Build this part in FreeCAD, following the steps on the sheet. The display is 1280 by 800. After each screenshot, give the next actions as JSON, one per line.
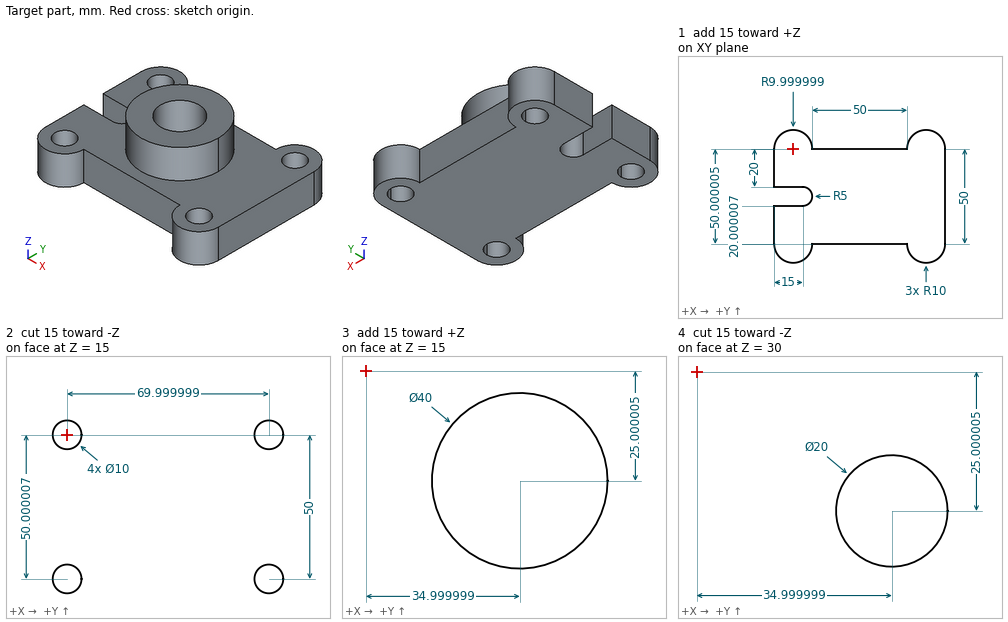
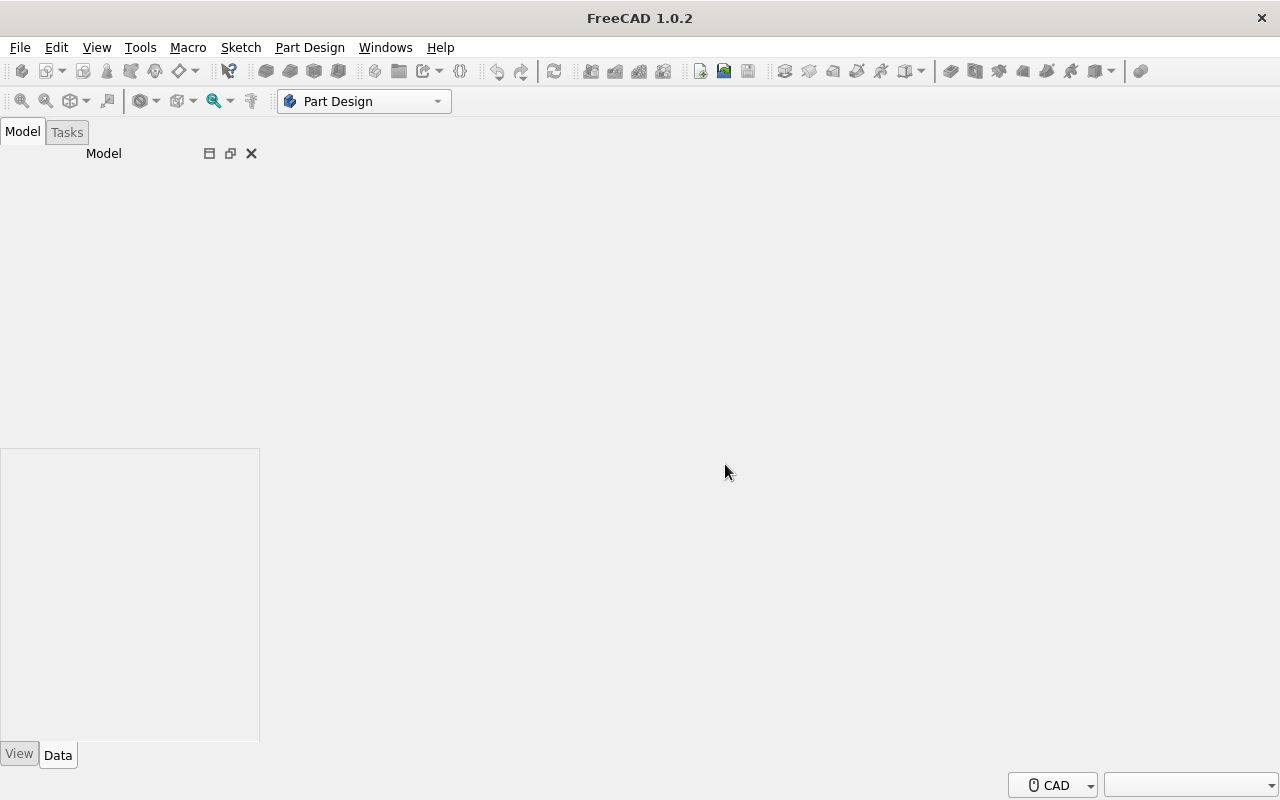
{"action": "left_click", "coordinate": [700, 72]}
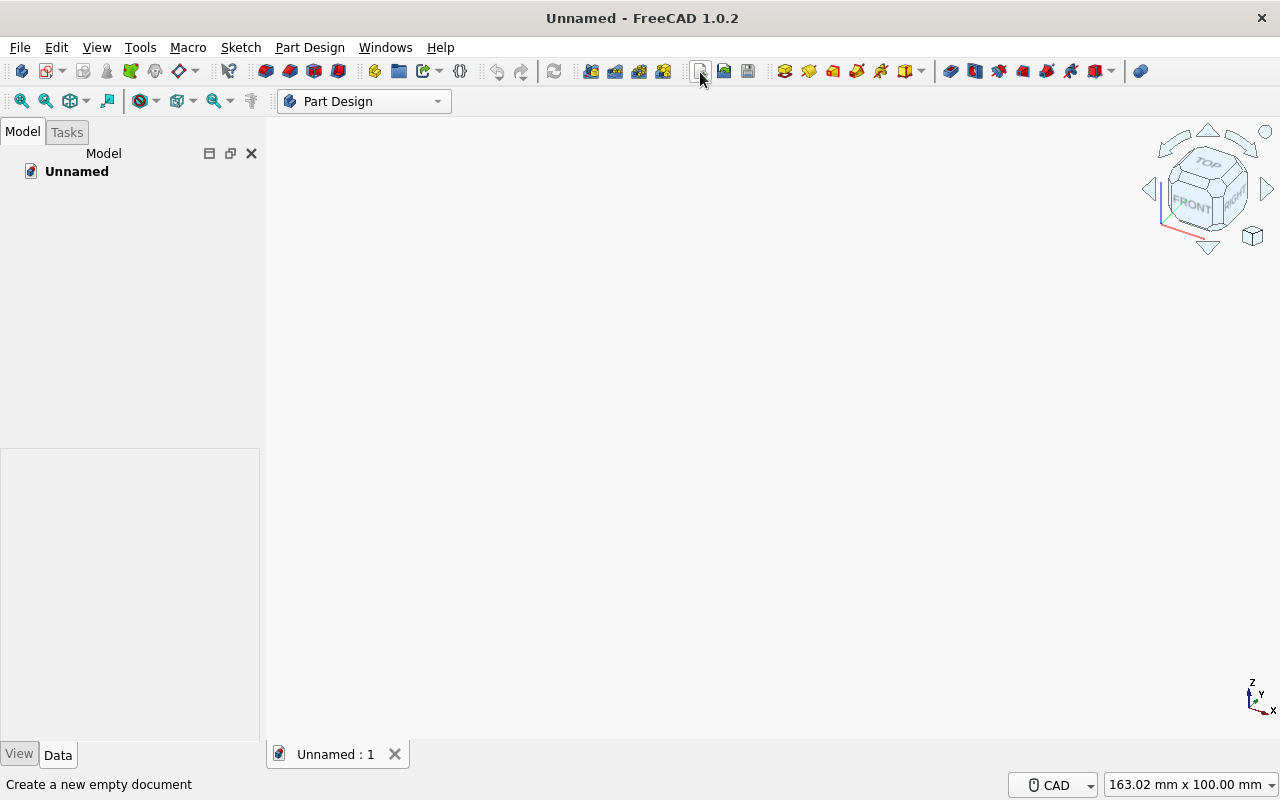
{"action": "left_click", "coordinate": [46, 72]}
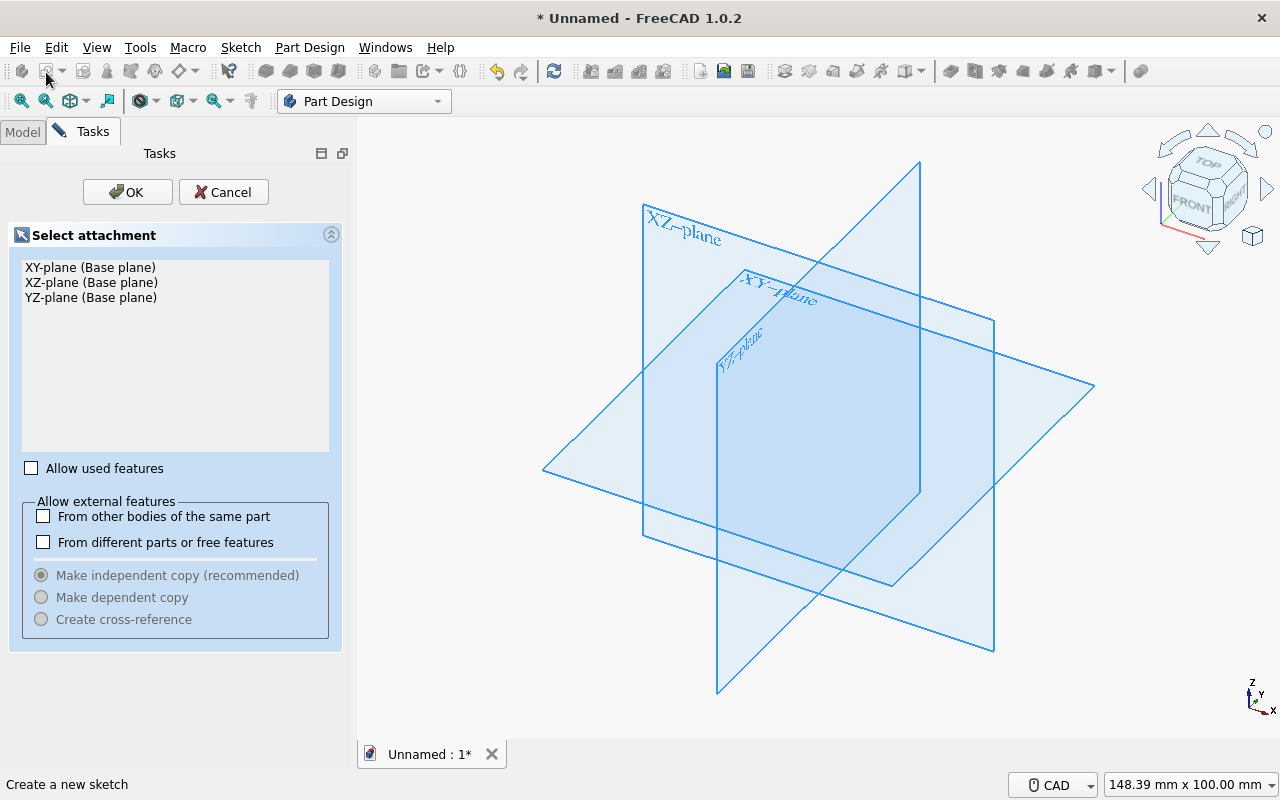
{"action": "left_click", "coordinate": [82, 268]}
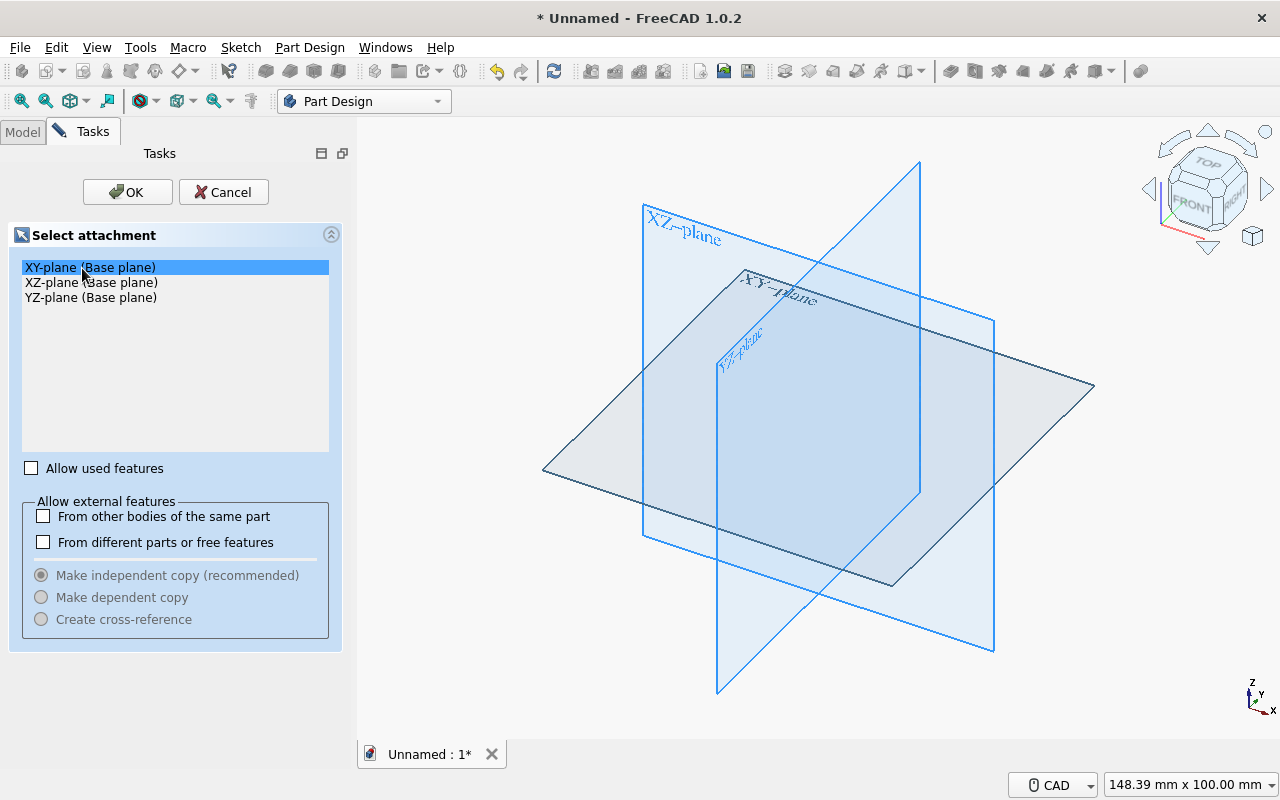
{"action": "left_click", "coordinate": [128, 192]}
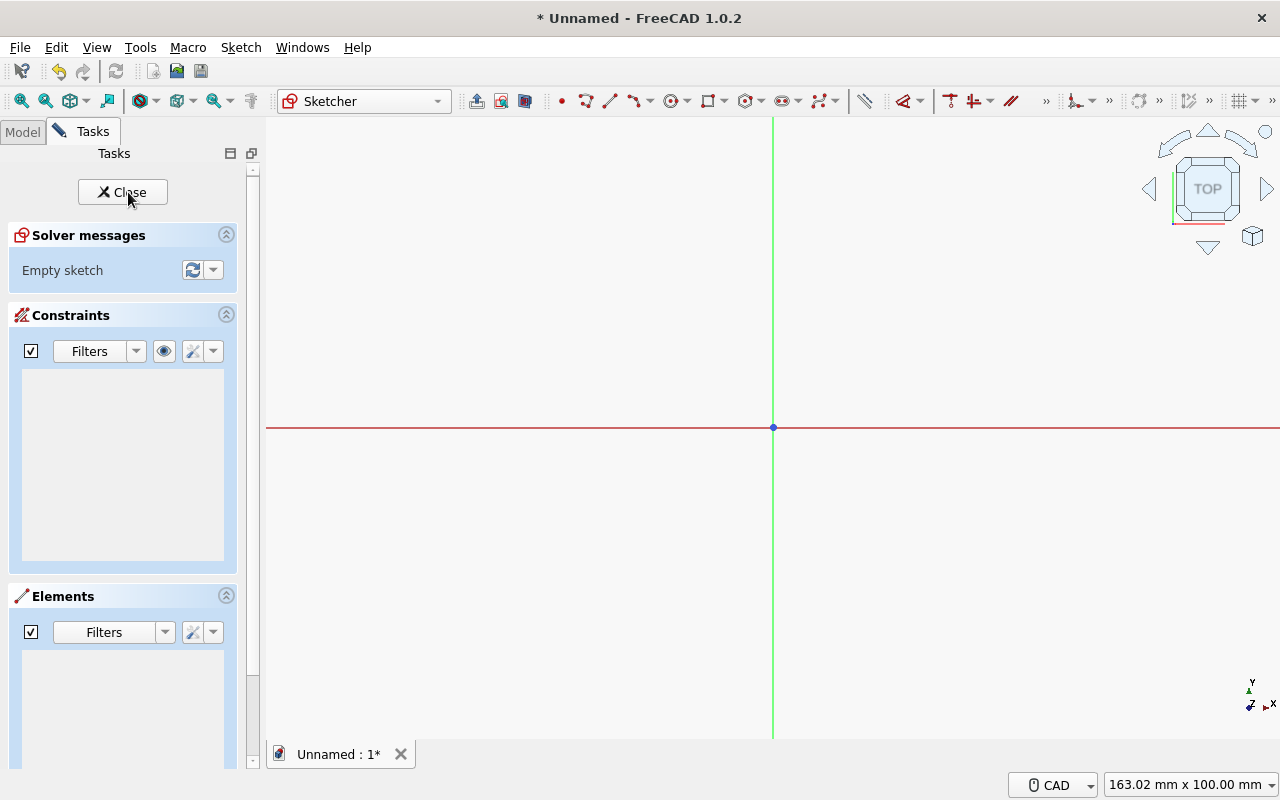
{"action": "scroll", "coordinate": [294, 145], "scroll_direction": "down", "scroll_amount": 2}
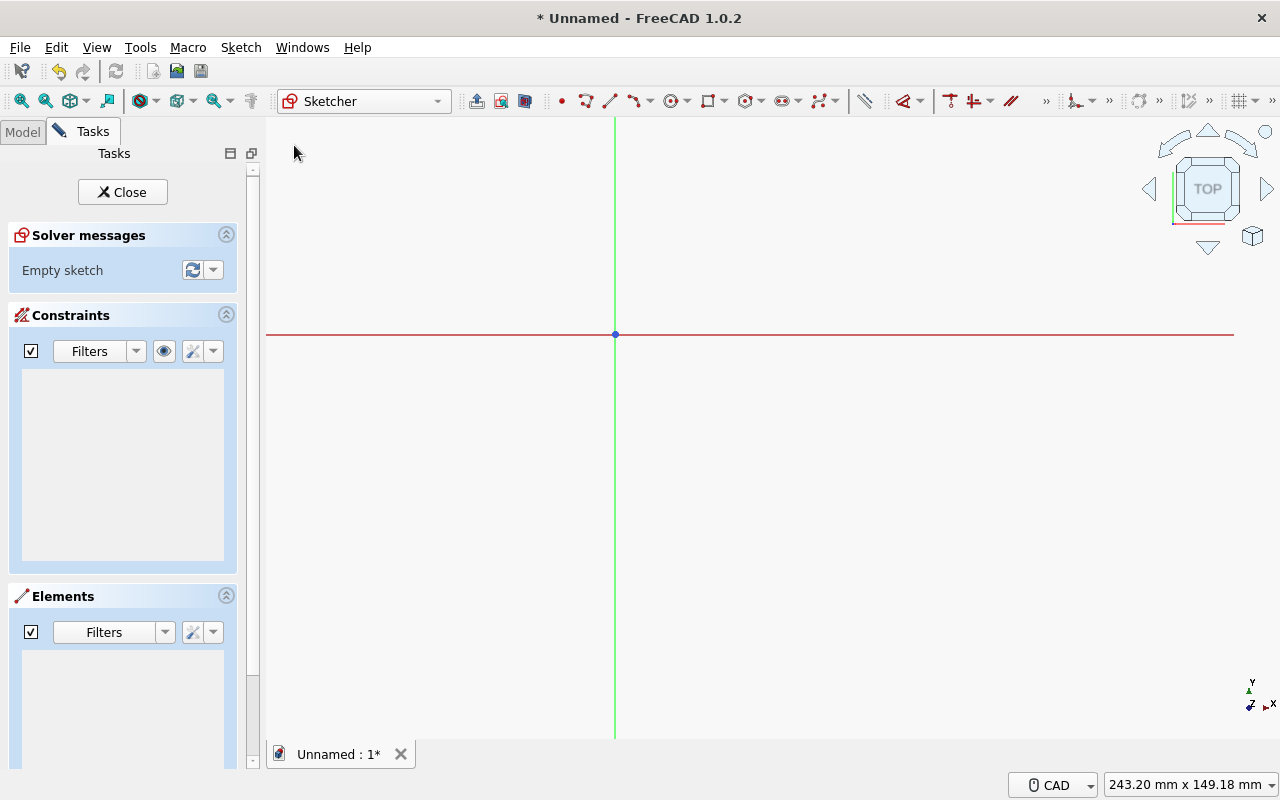
{"action": "scroll", "coordinate": [876, 461], "scroll_direction": "up", "scroll_amount": 2}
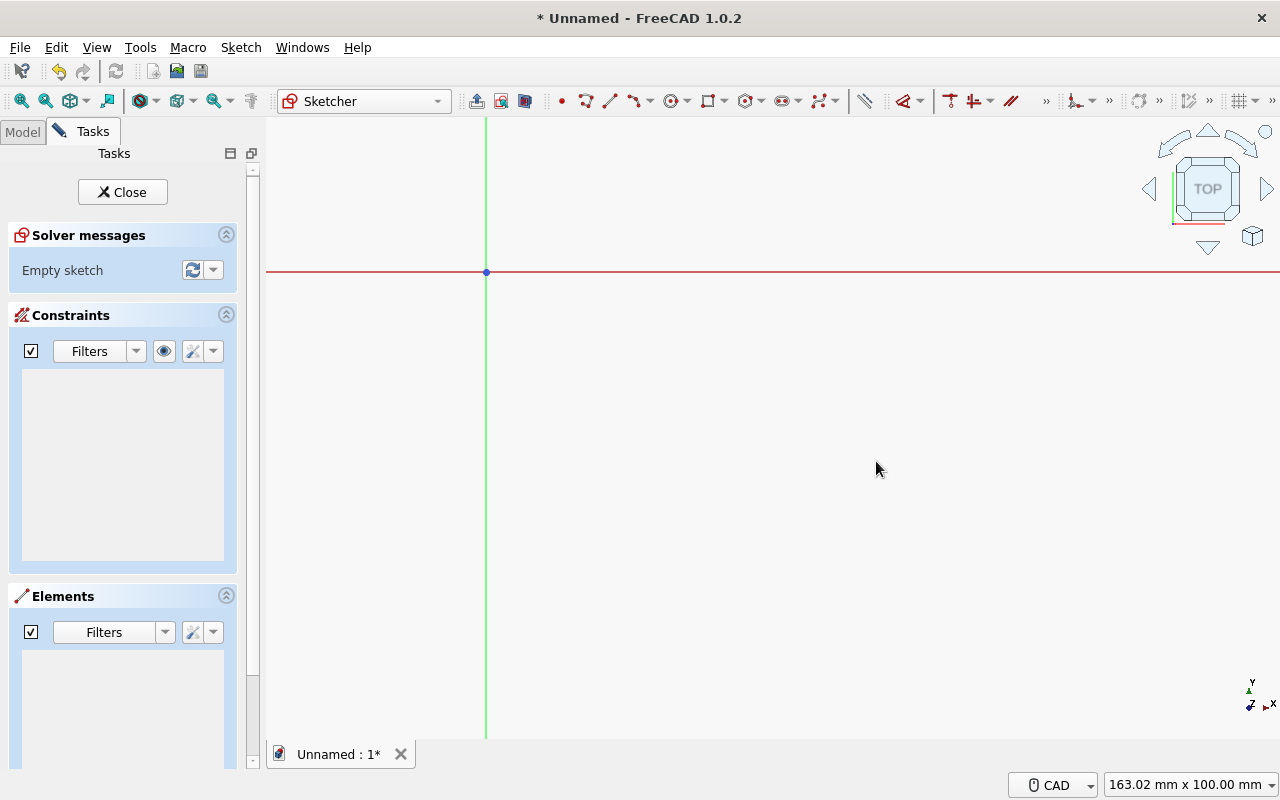
{"action": "left_click", "coordinate": [610, 102]}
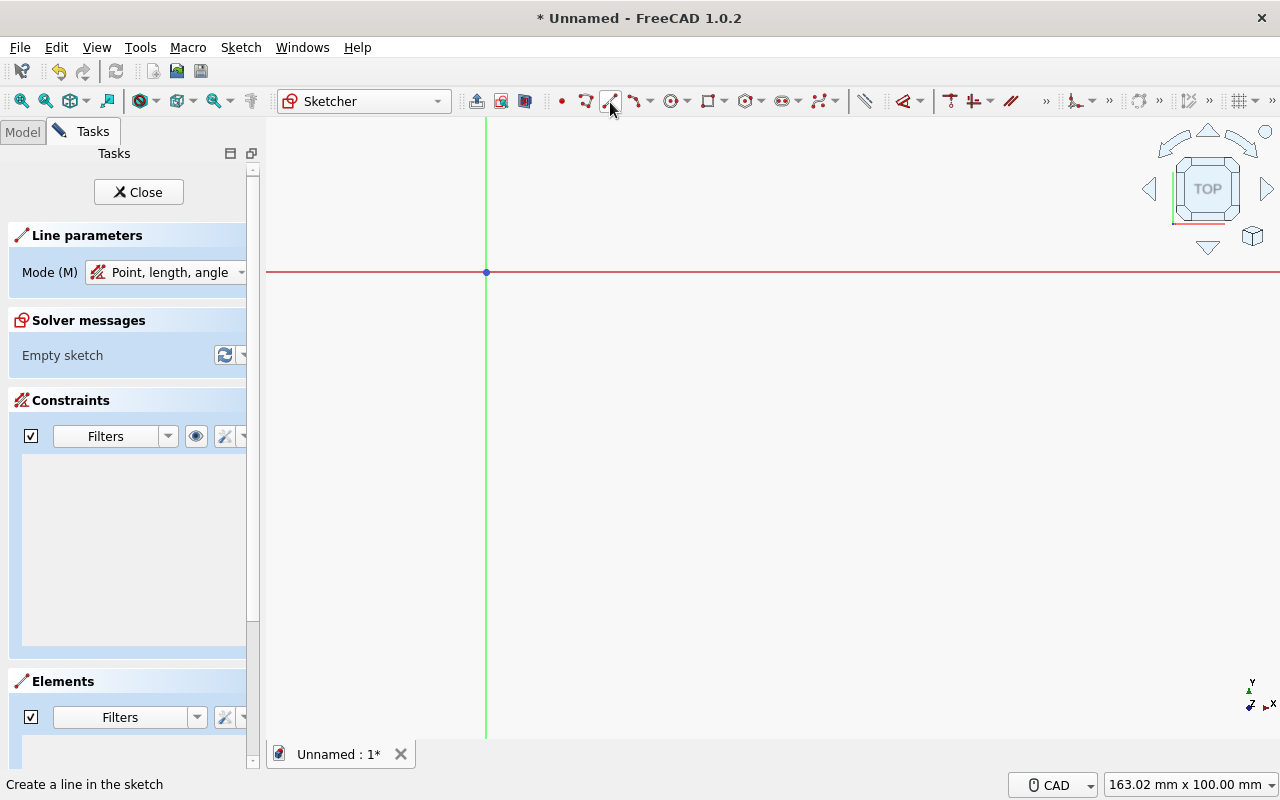
{"action": "left_click", "coordinate": [860, 272]}
{"action": "left_click", "coordinate": [549, 281]}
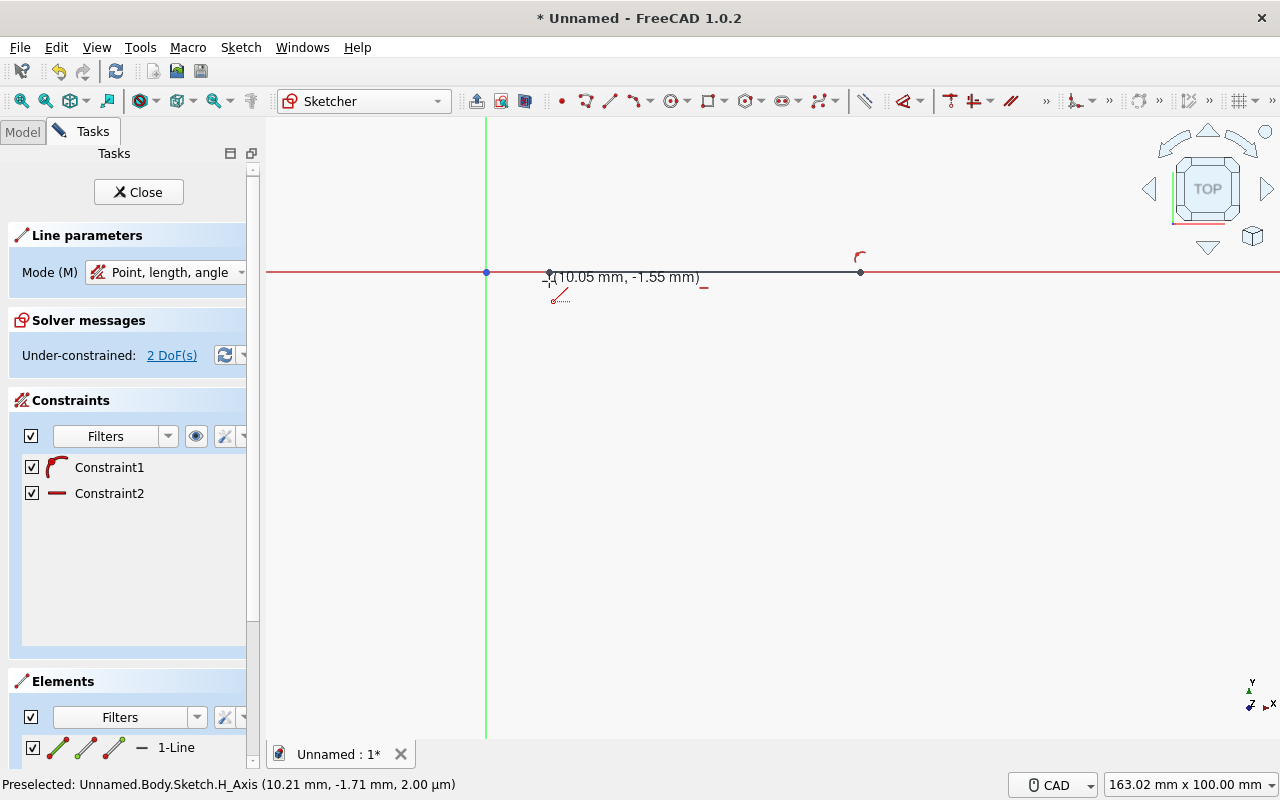
{"action": "left_click", "coordinate": [586, 102]}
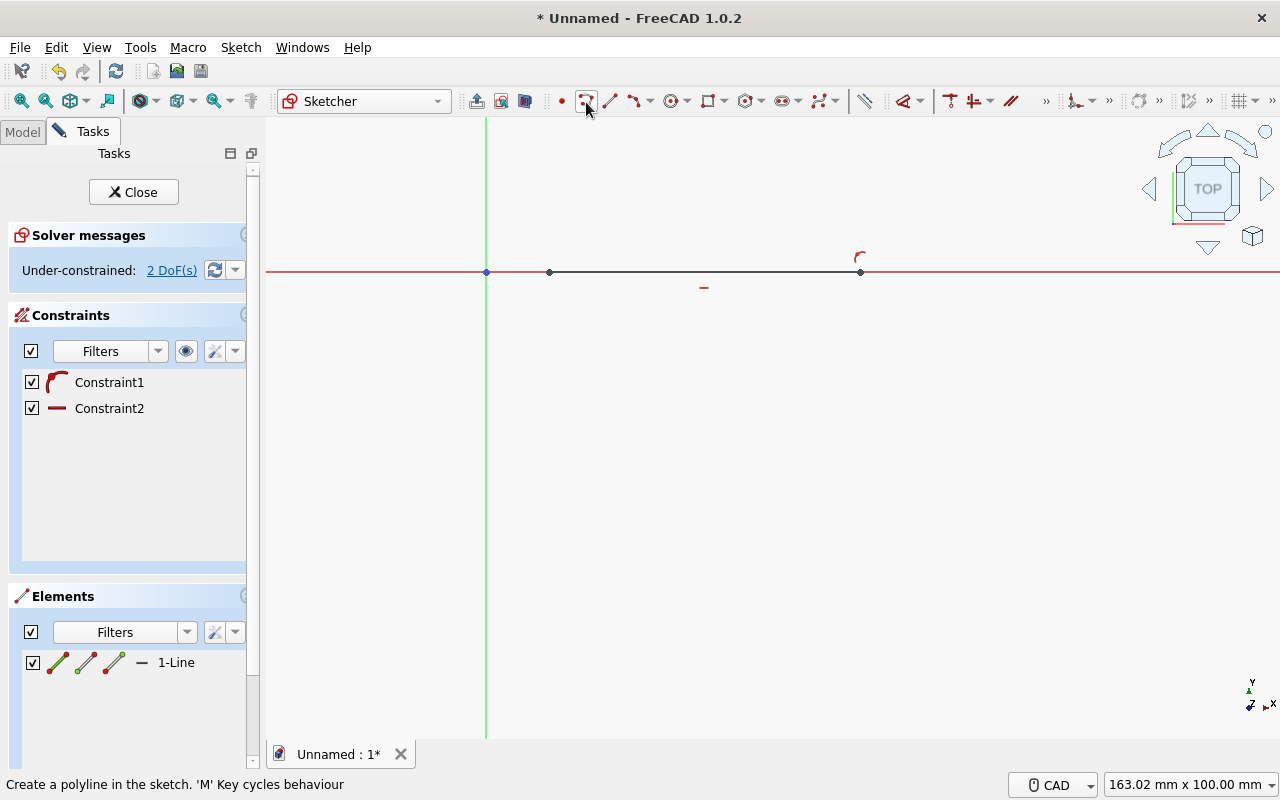
{"action": "left_click", "coordinate": [424, 272]}
{"action": "left_click", "coordinate": [424, 397]}
{"action": "left_click", "coordinate": [518, 397]}
{"action": "right_click", "coordinate": [518, 397]}